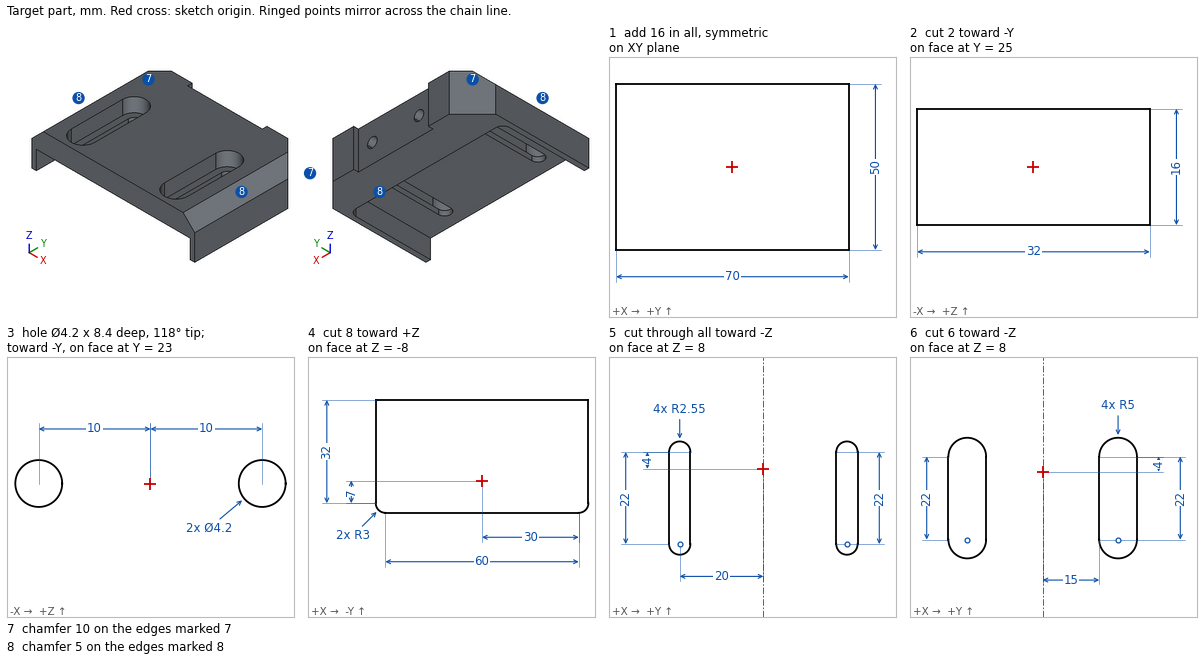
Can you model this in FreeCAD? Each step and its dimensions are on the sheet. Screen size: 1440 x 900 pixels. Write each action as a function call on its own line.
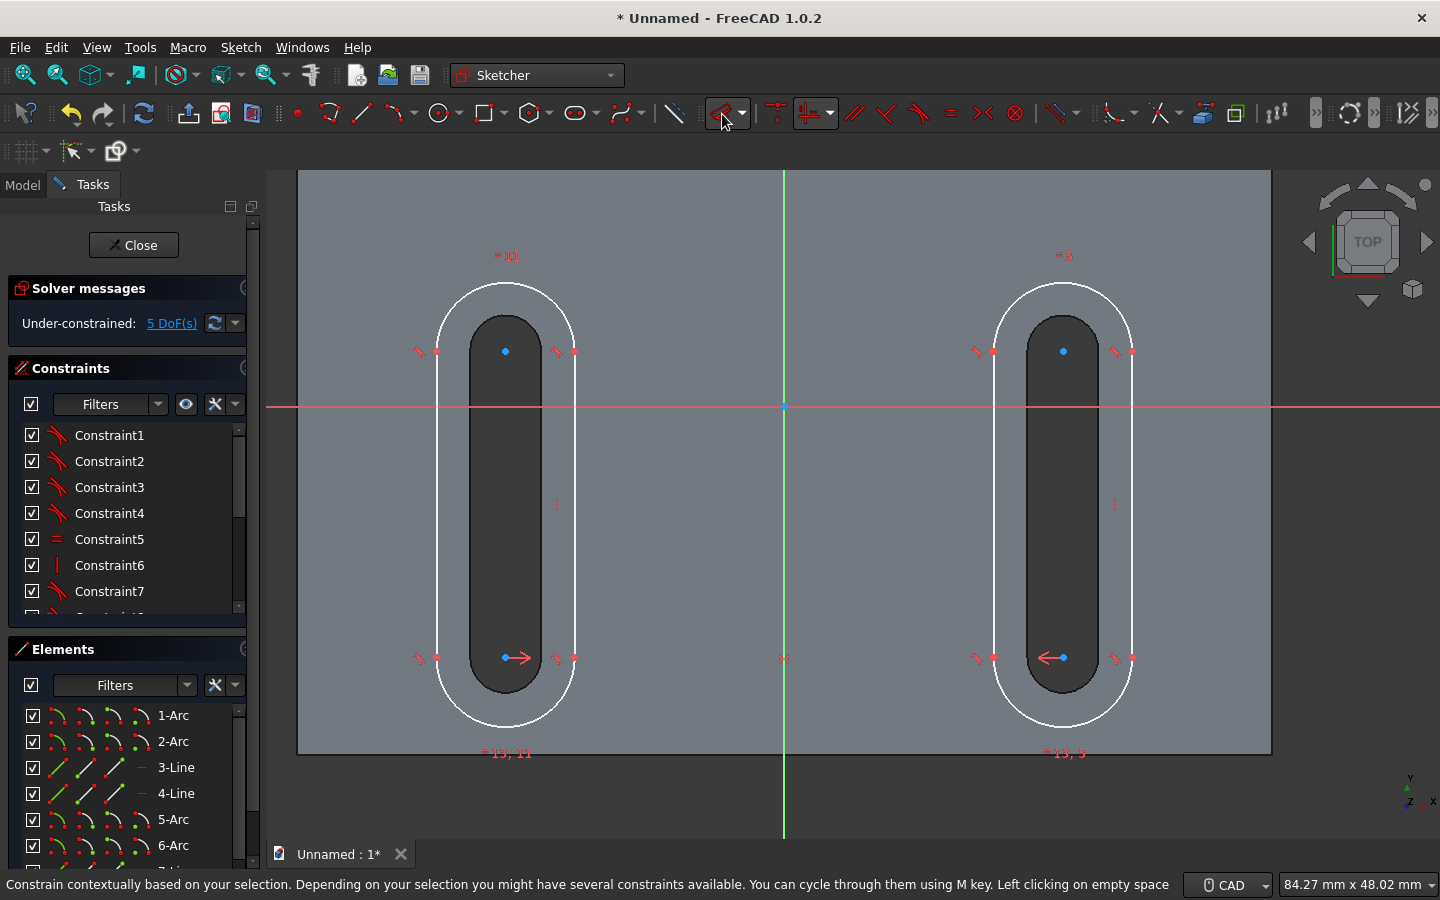
click(1022, 714)
click(1003, 740)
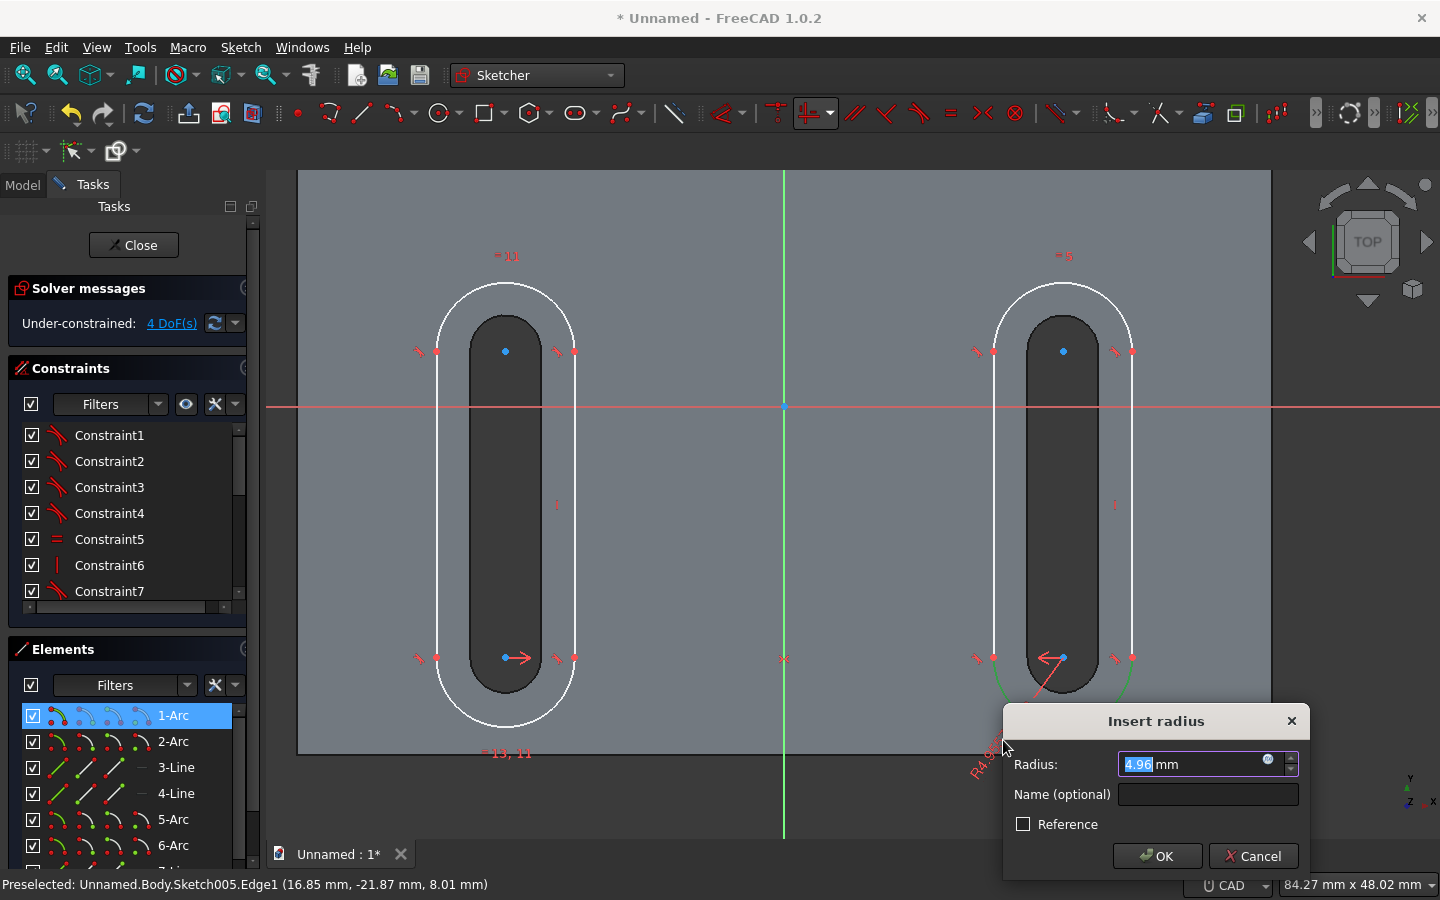
text(5)
key(Return)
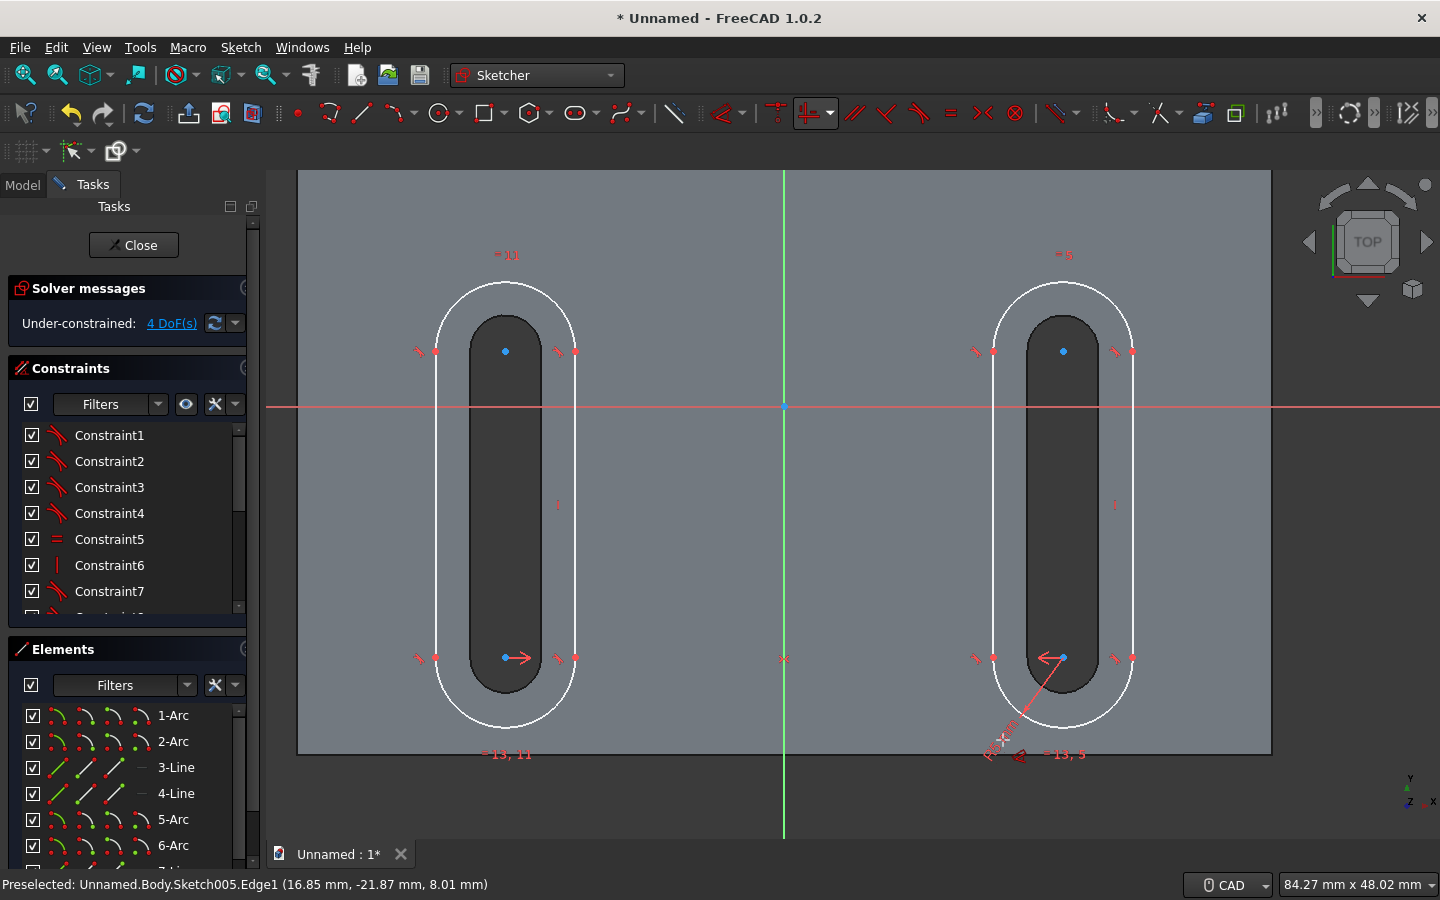
click(993, 566)
click(1027, 505)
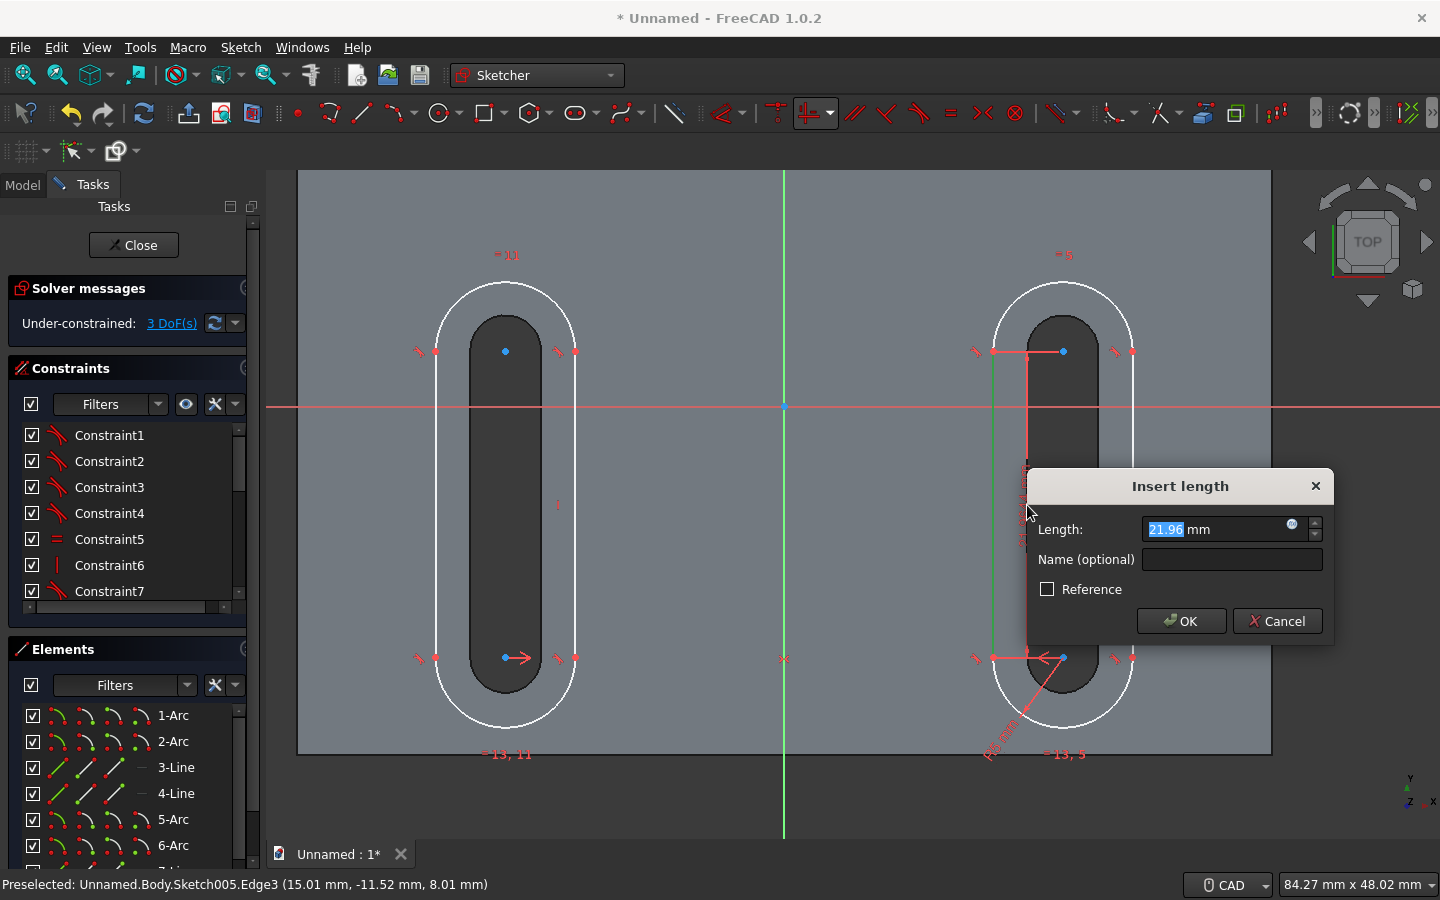
text(22)
key(Return)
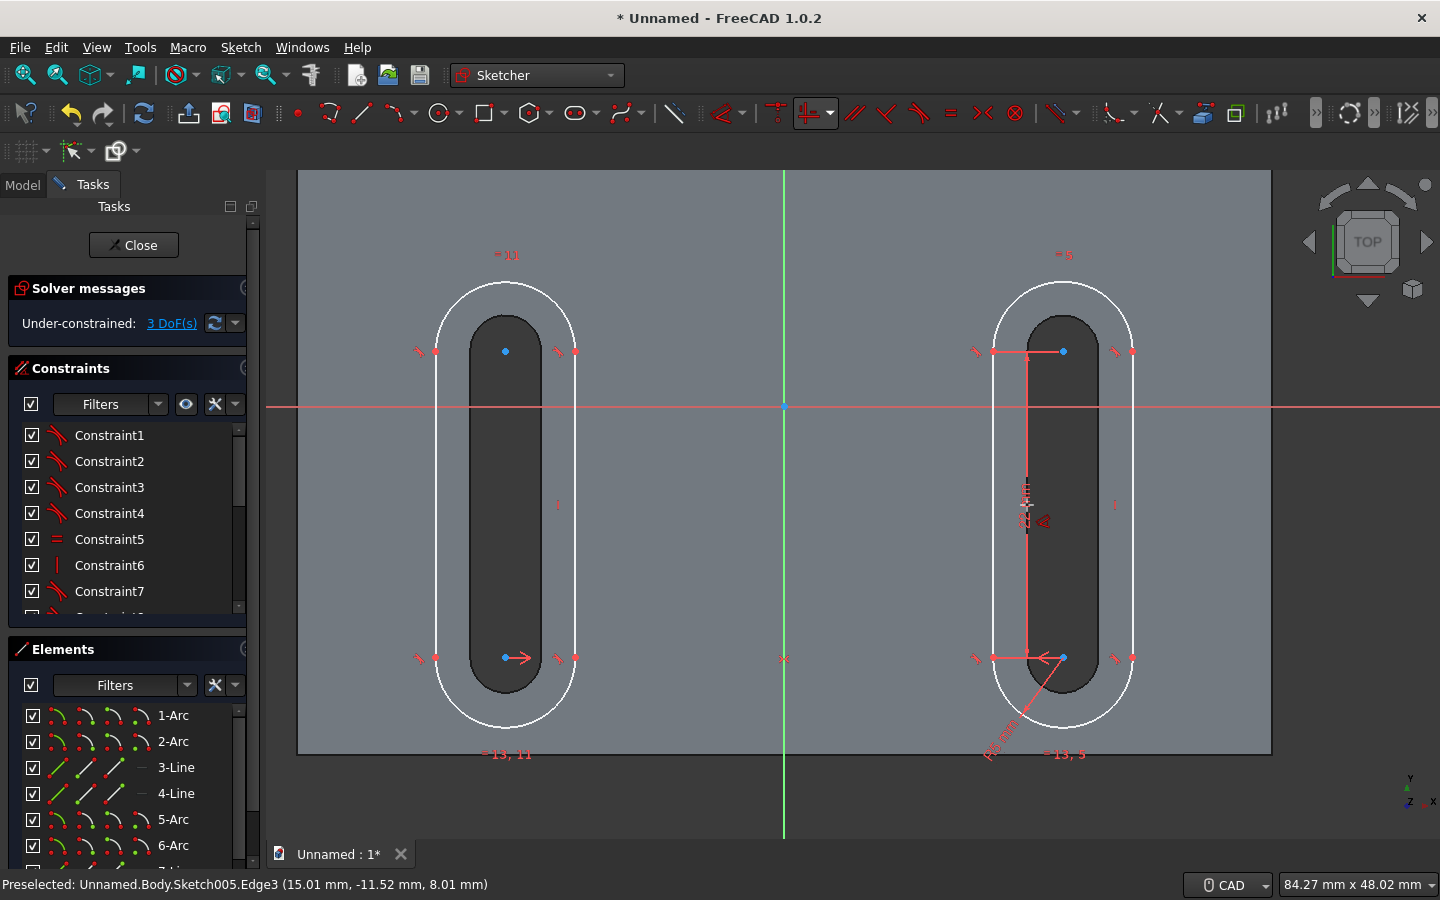
click(436, 566)
click(402, 505)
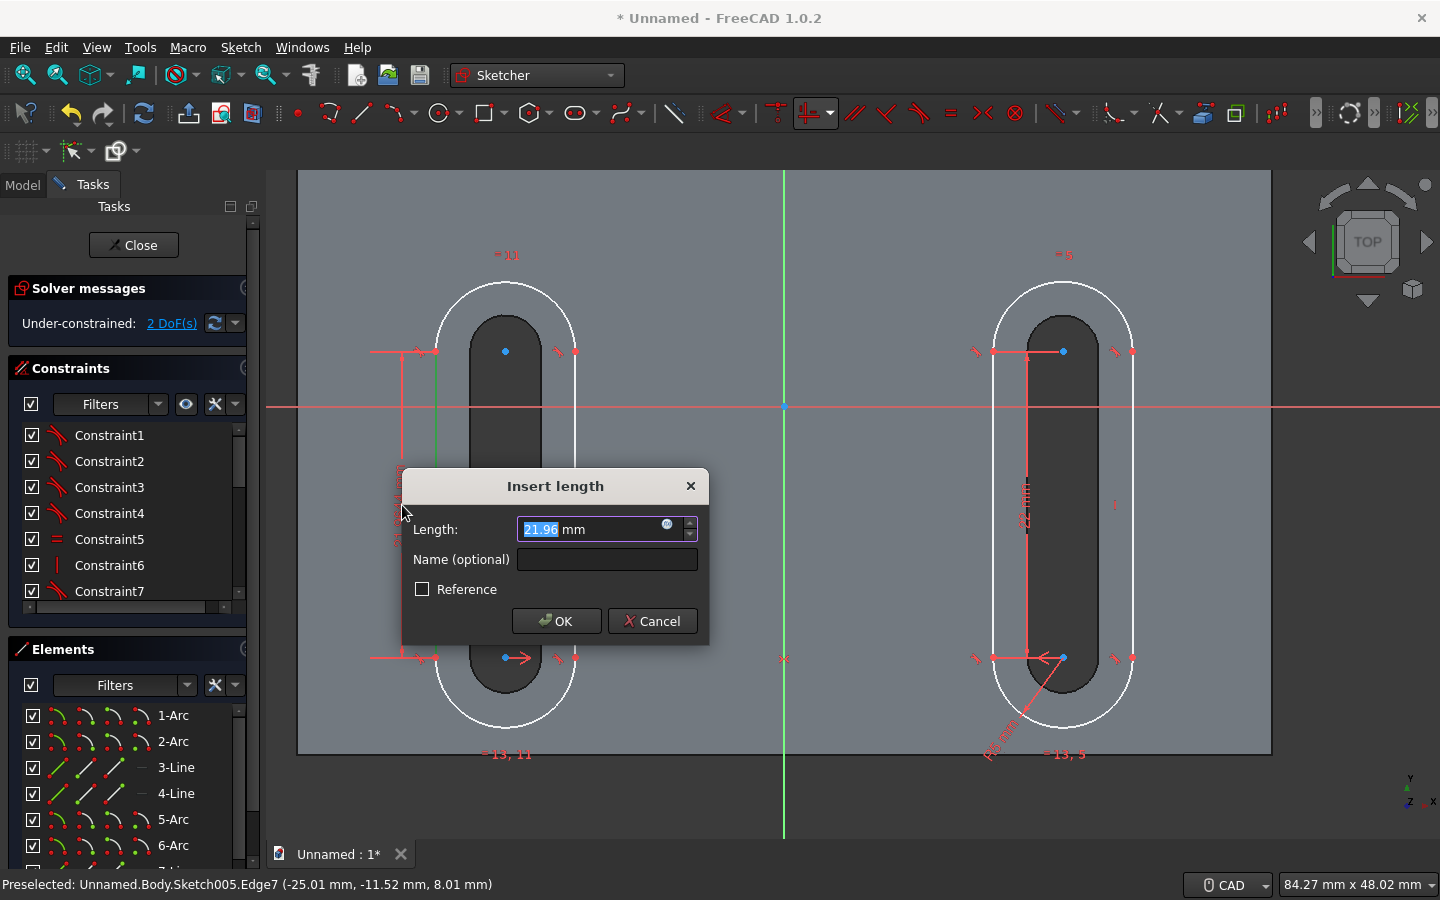
text(22)
key(Return)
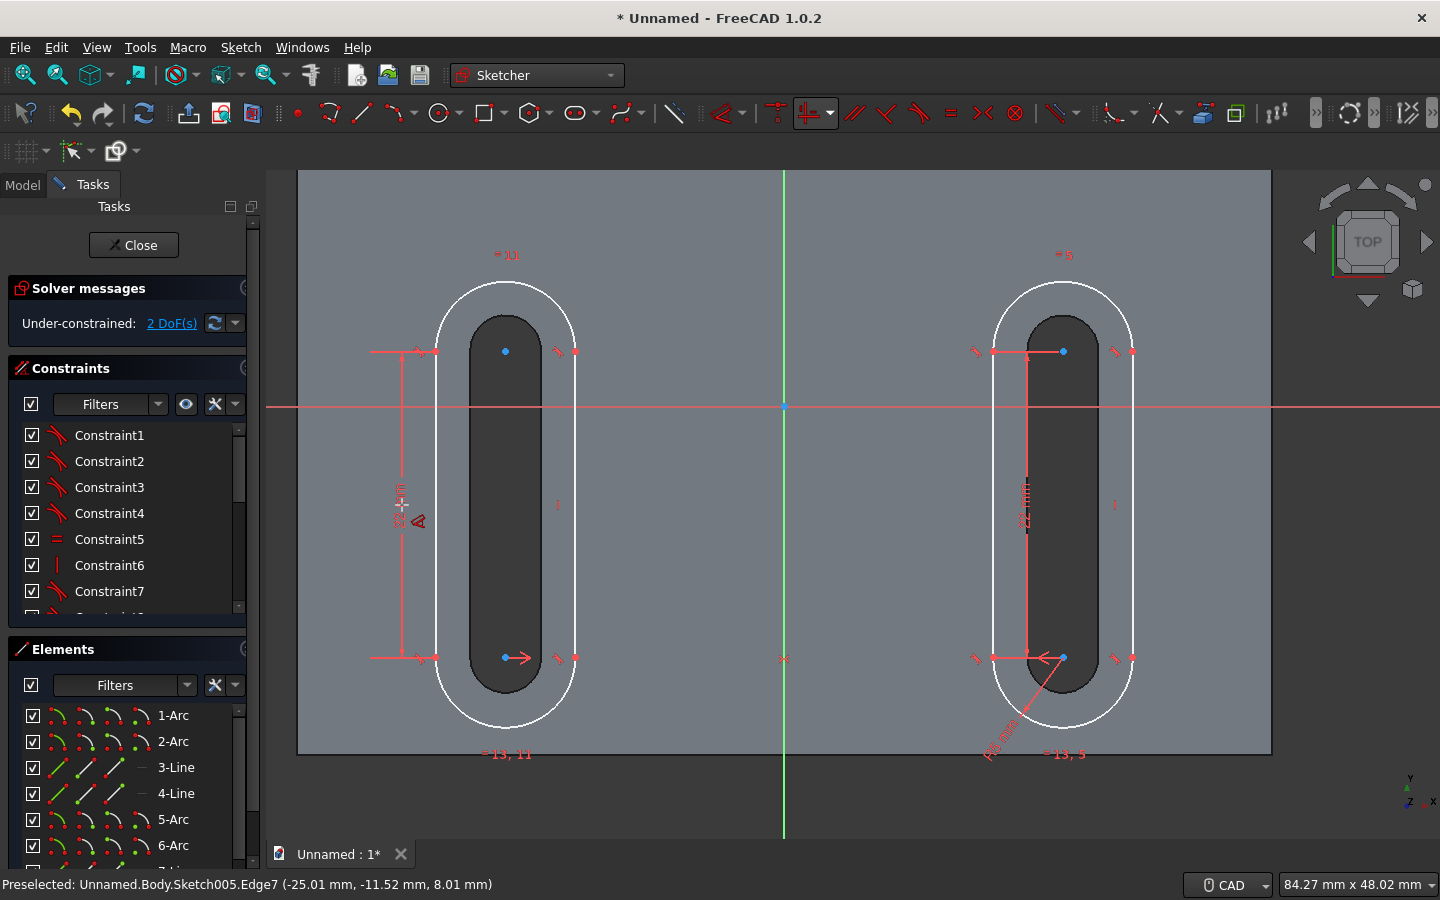
click(1133, 352)
click(1167, 379)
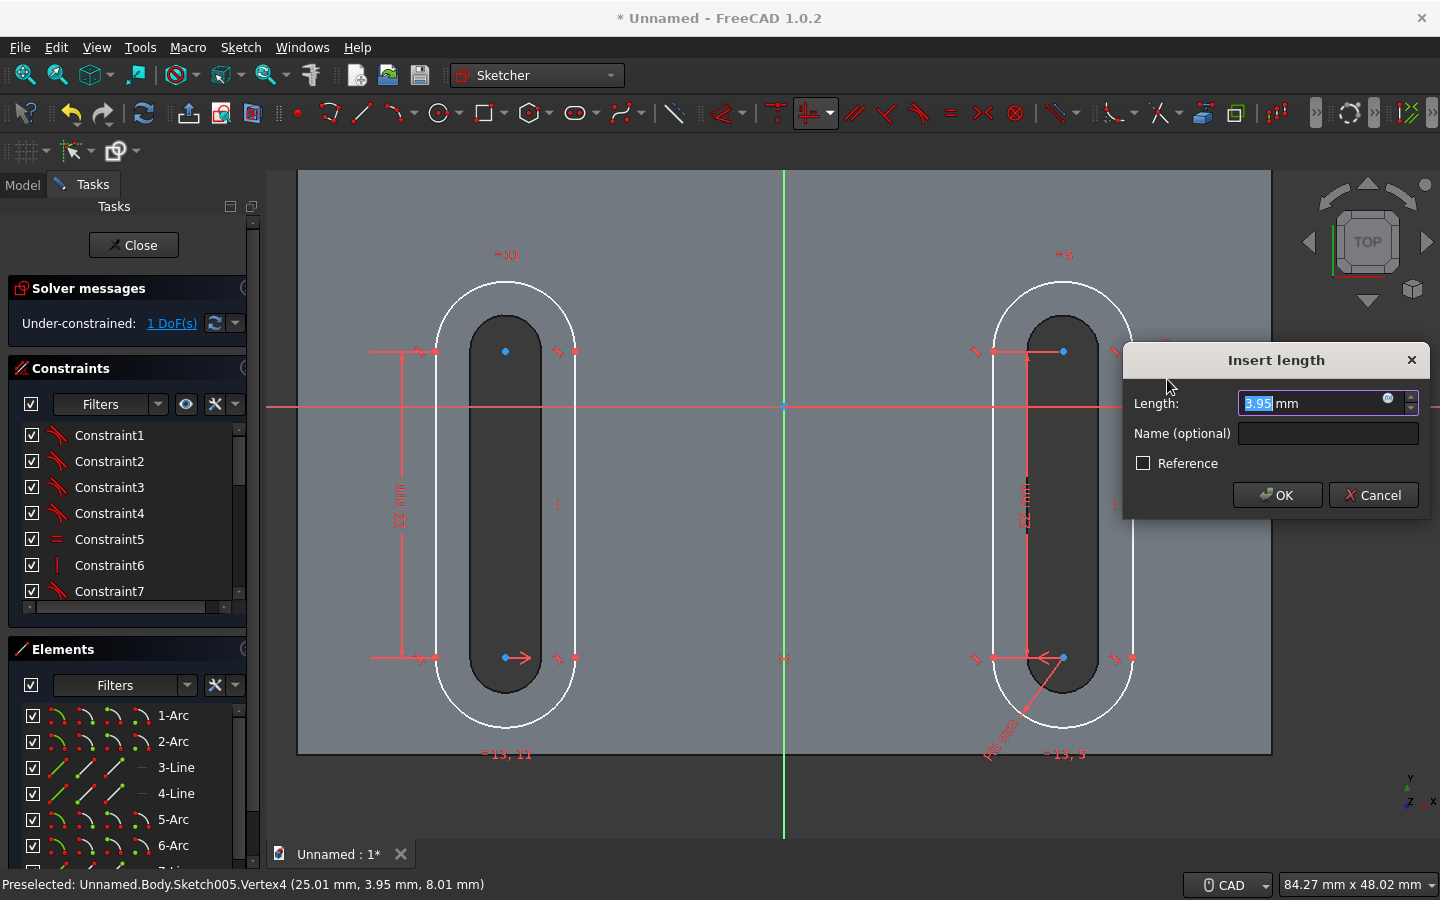
text(4)
key(Return)